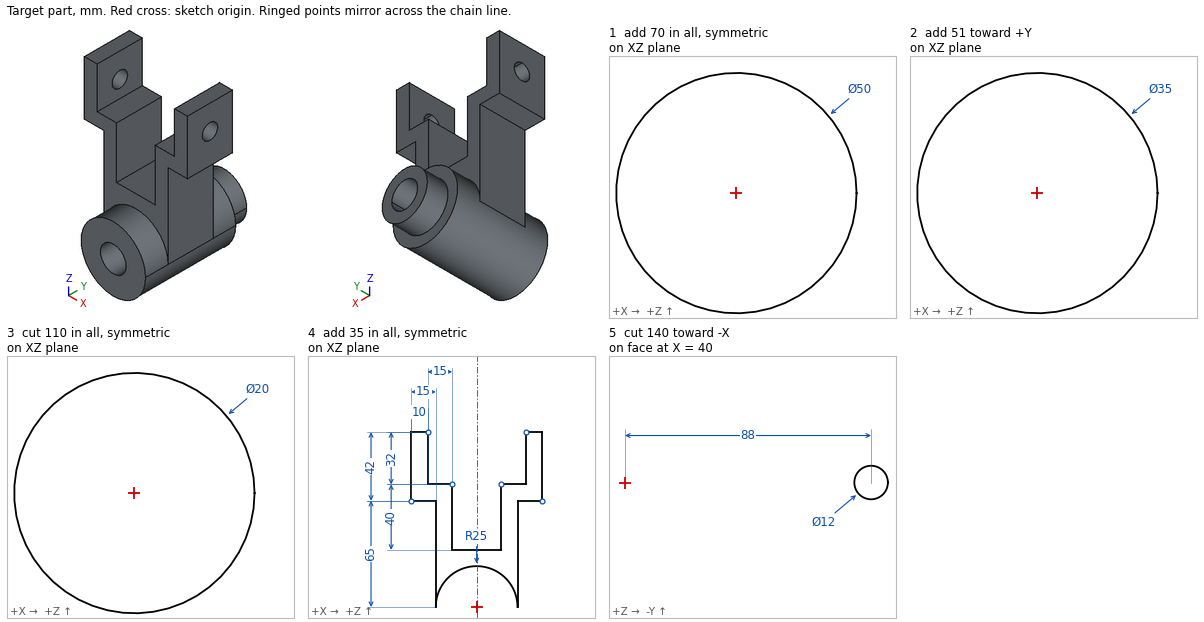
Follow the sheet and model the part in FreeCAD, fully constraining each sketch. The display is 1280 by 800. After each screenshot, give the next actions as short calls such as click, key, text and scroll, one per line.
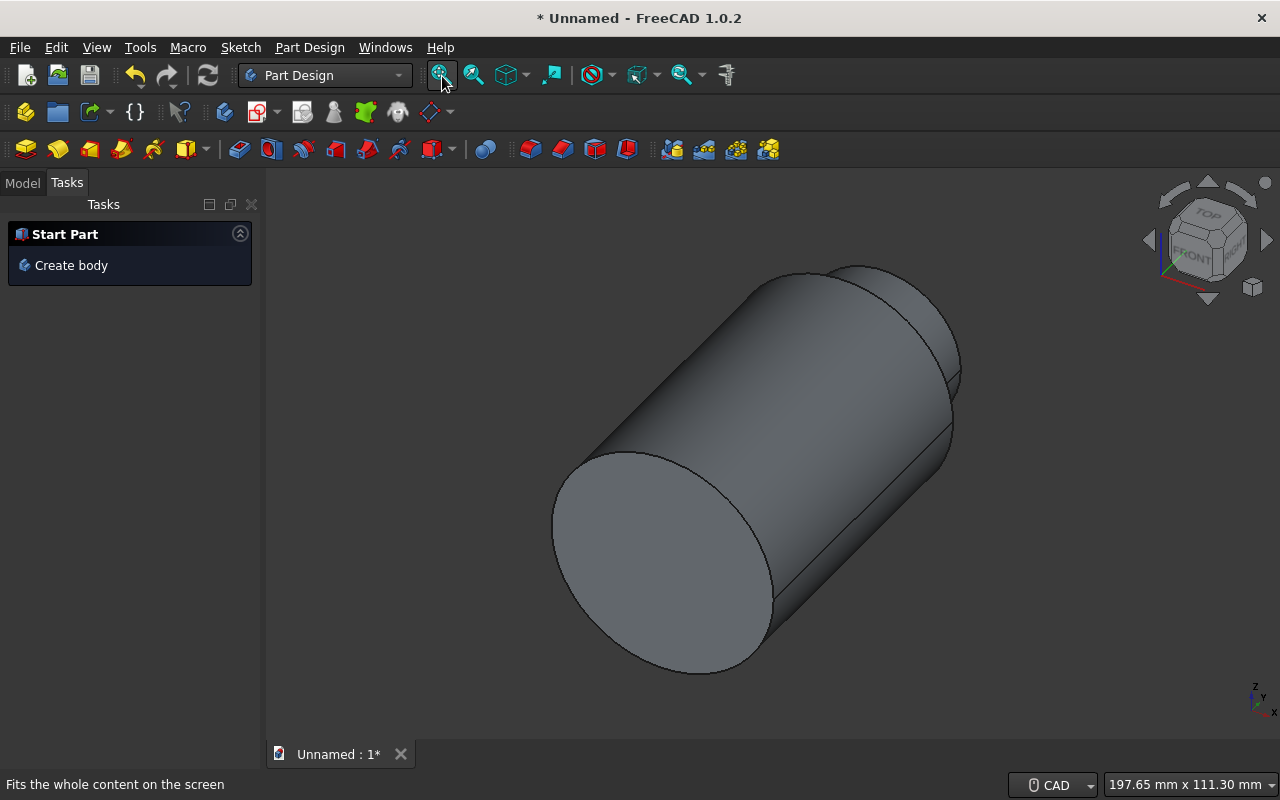
click(258, 112)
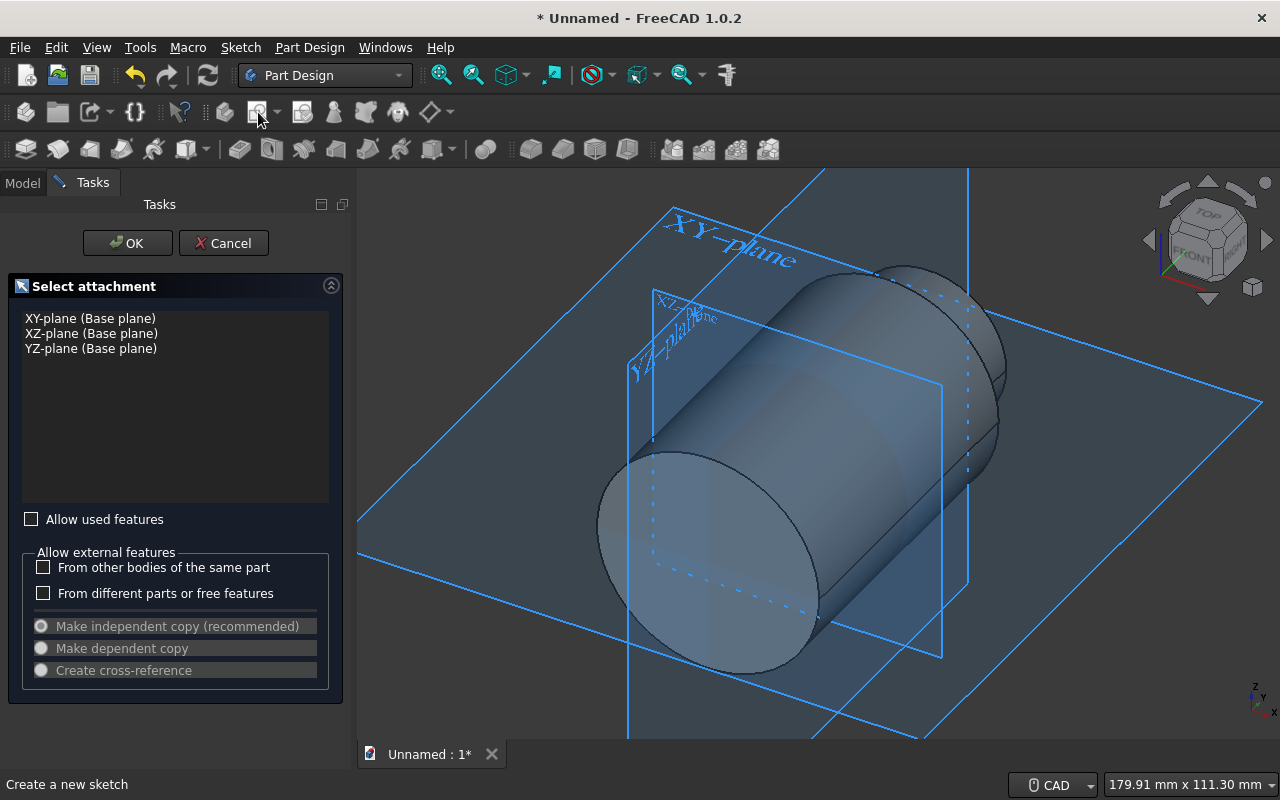
click(82, 334)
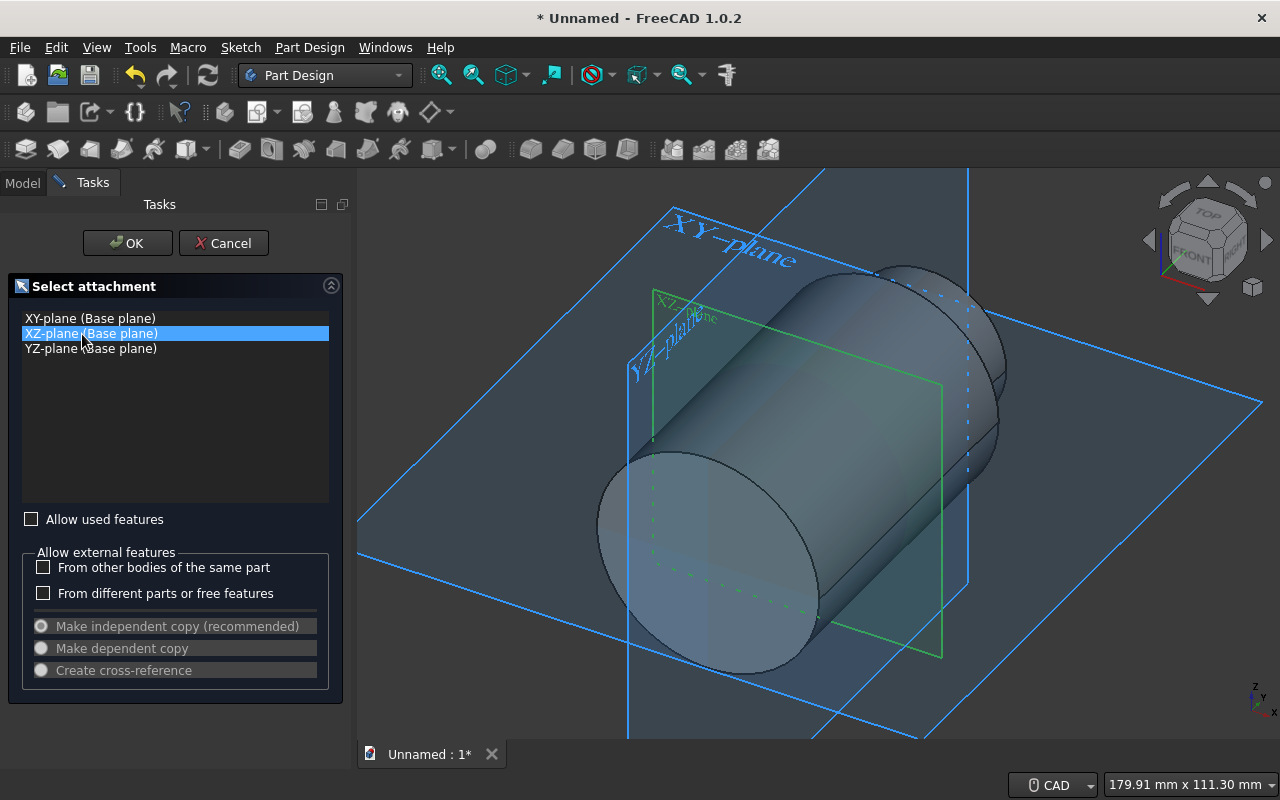
click(128, 243)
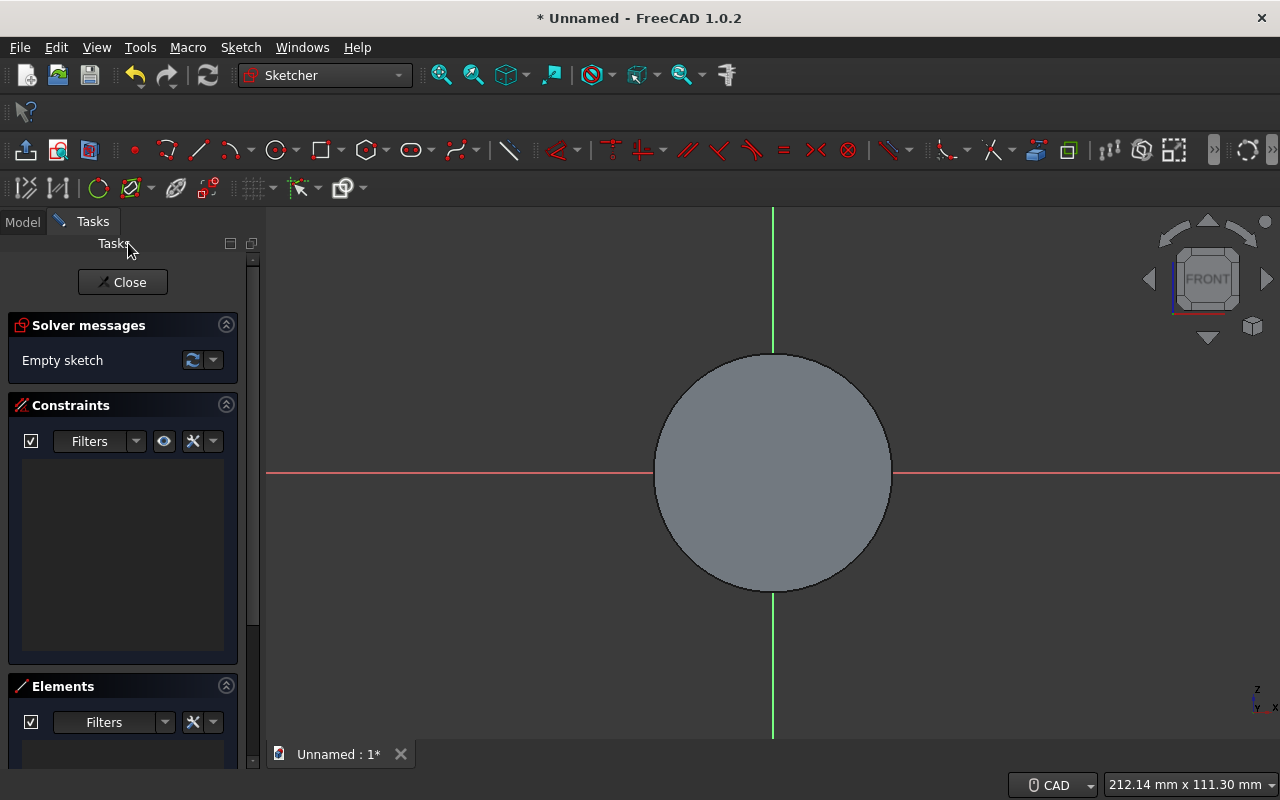
click(90, 150)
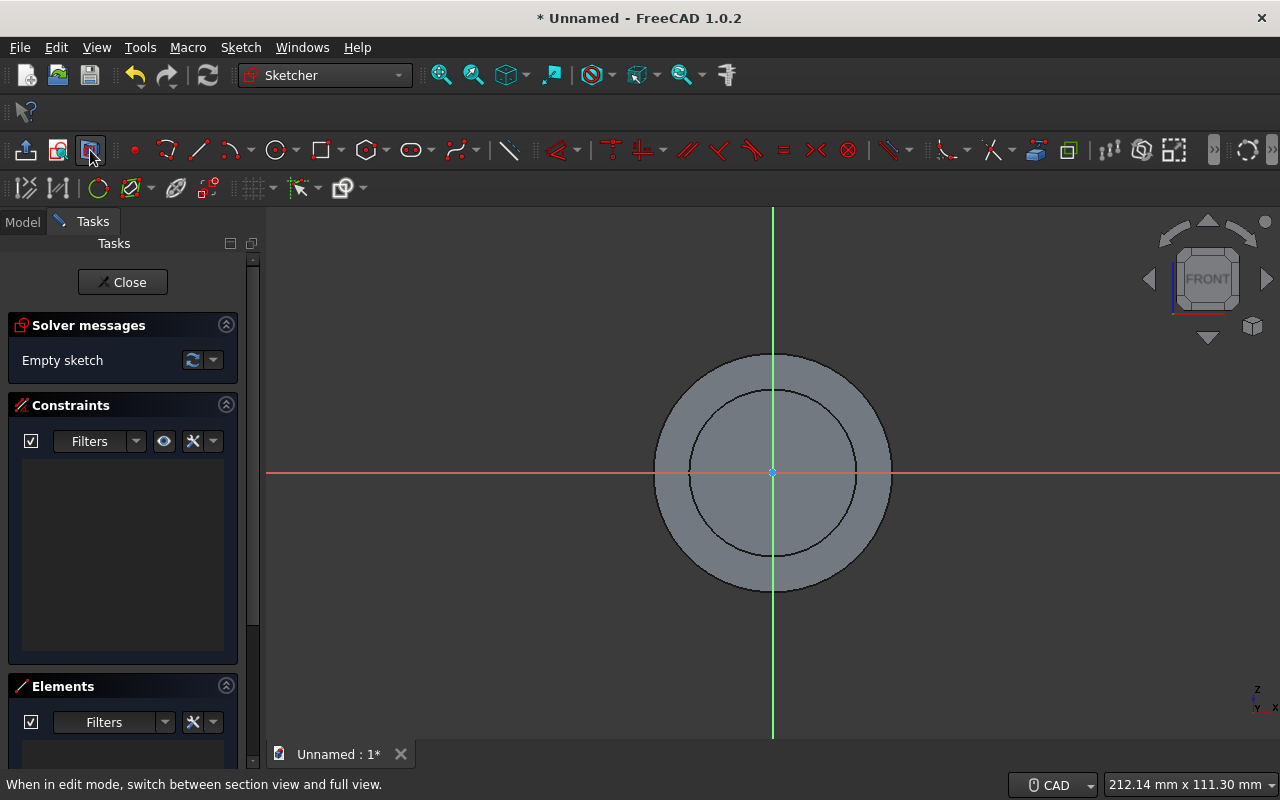
scroll(802, 473, up, 6)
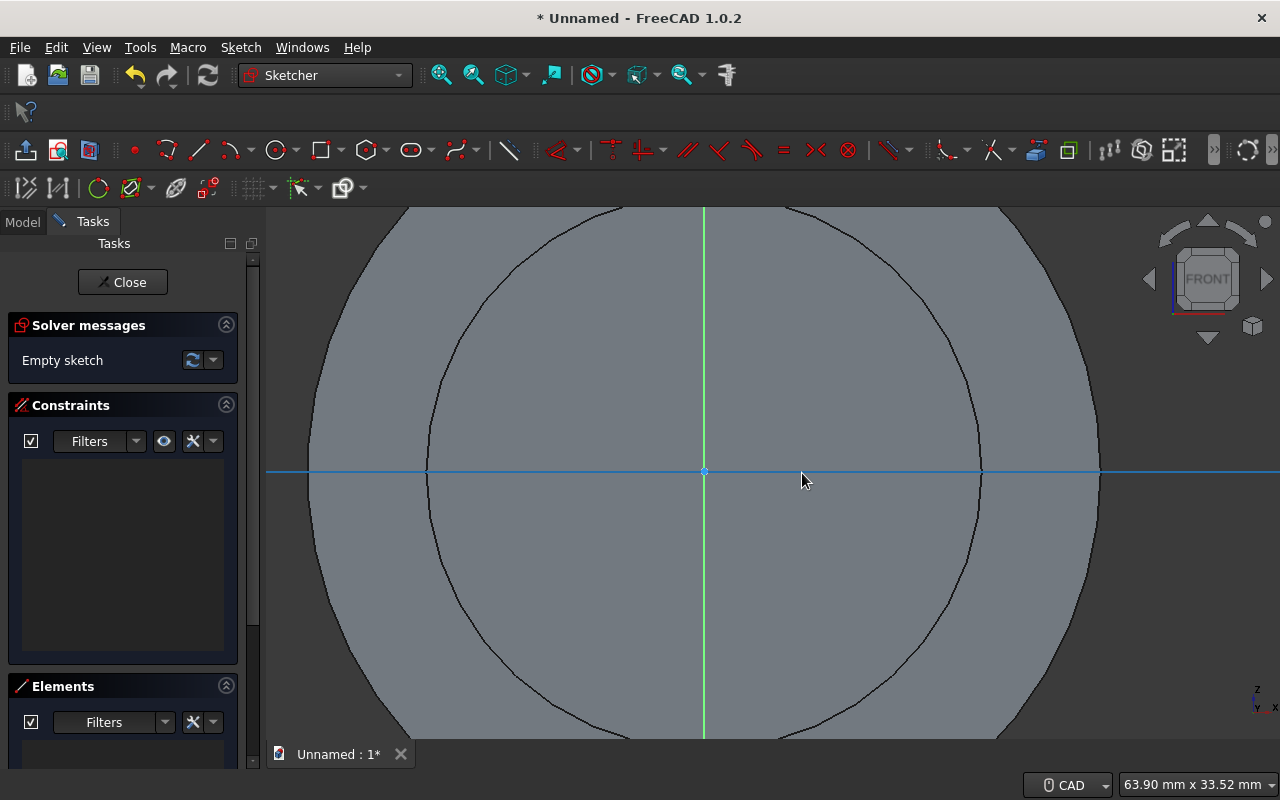
key(g)
key(c)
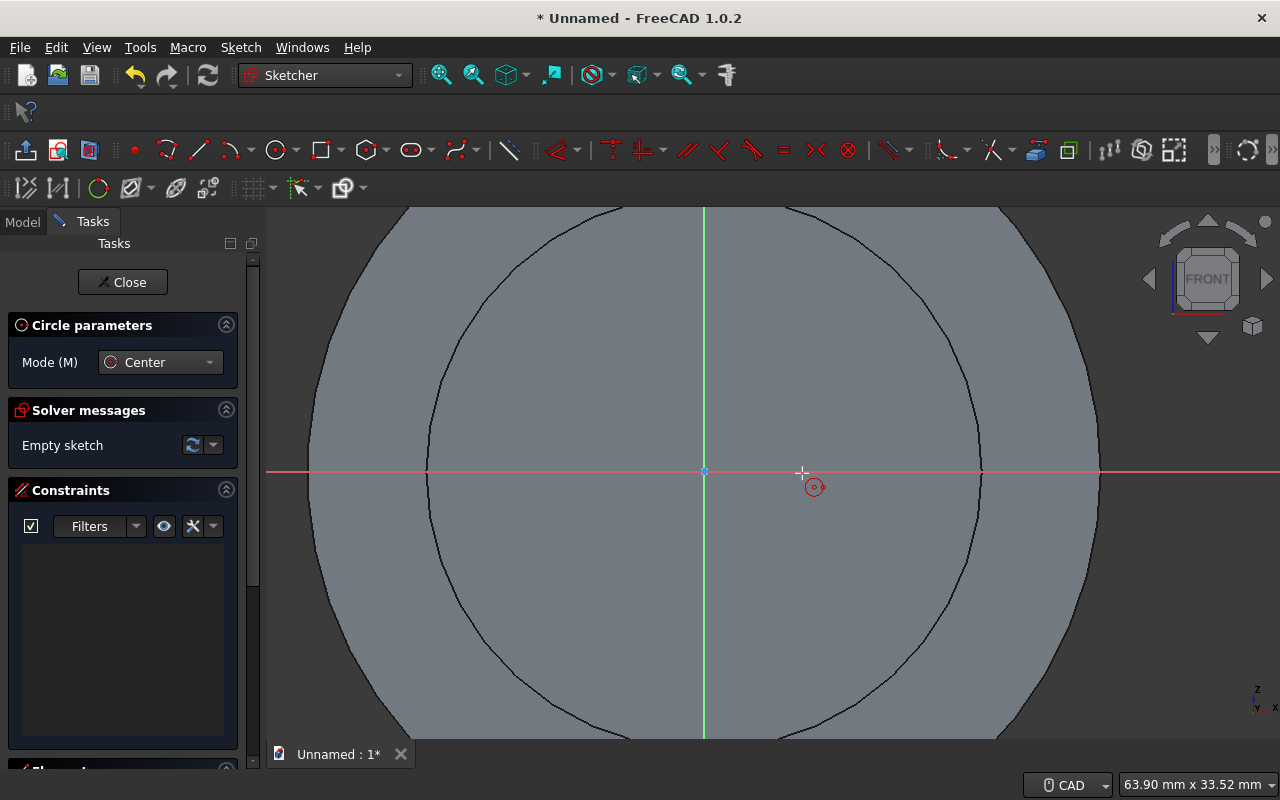
click(704, 472)
click(816, 360)
key(Escape)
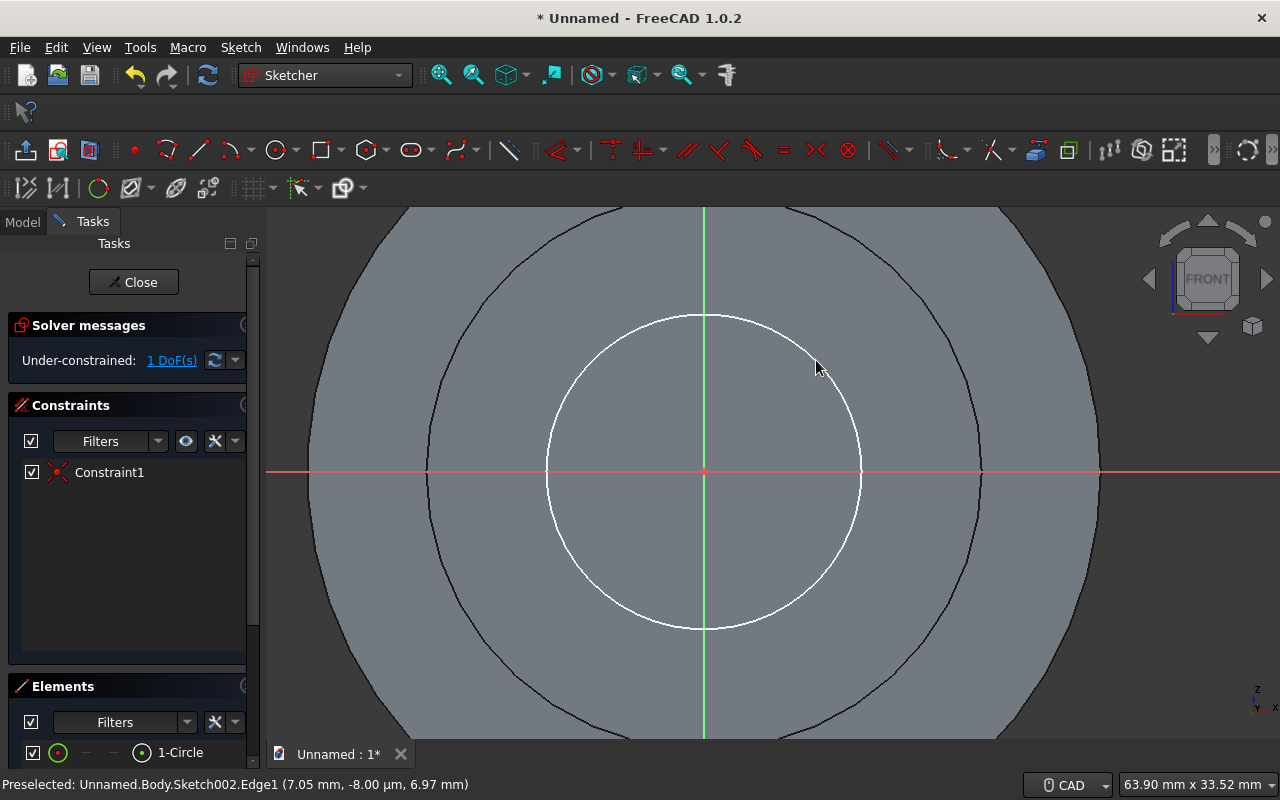
click(556, 150)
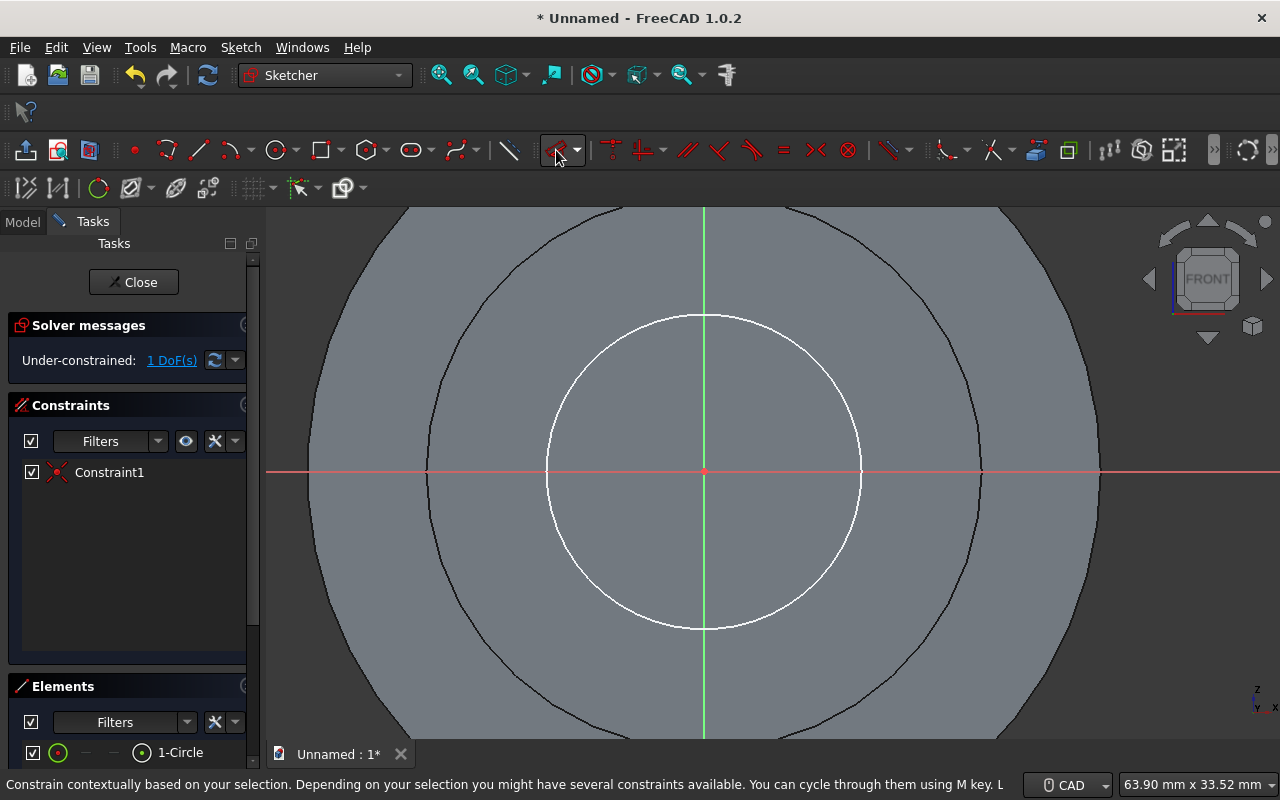
click(815, 360)
click(838, 337)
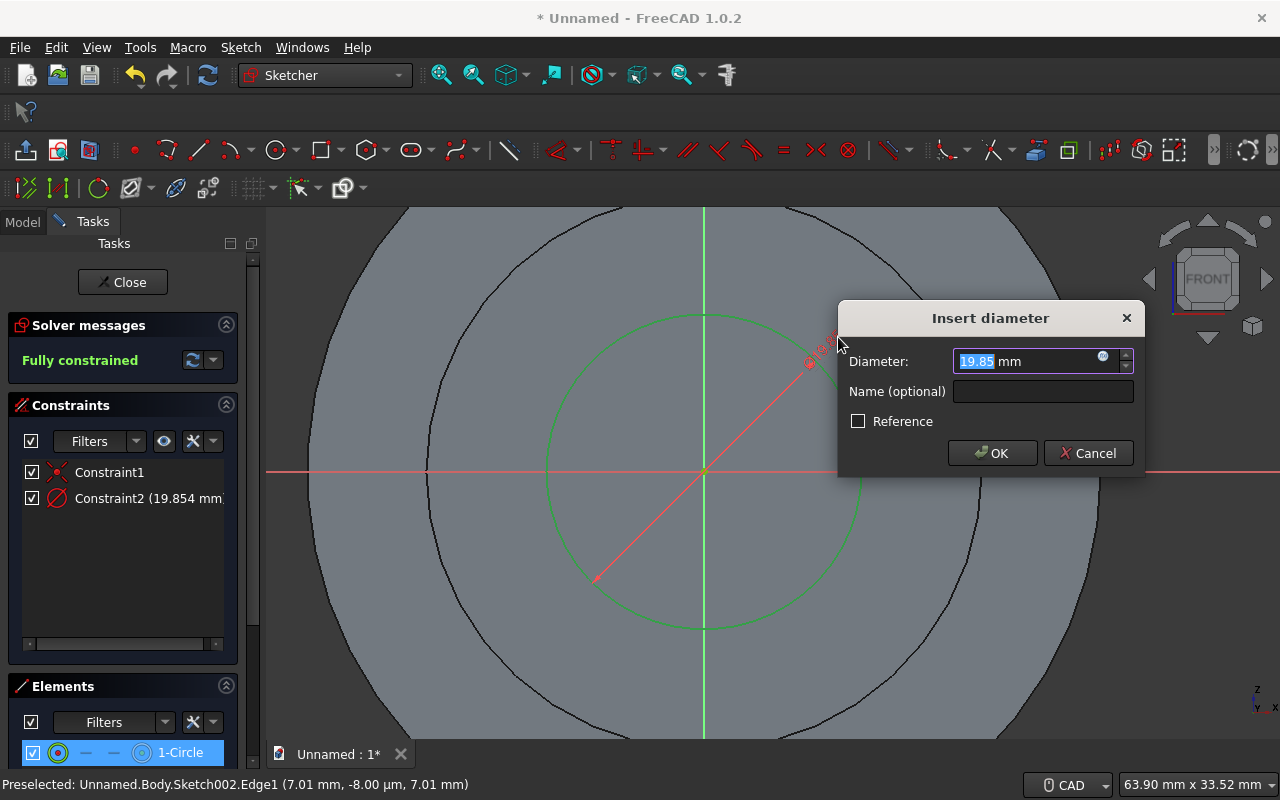
text(20)
key(Return)
key(Escape)